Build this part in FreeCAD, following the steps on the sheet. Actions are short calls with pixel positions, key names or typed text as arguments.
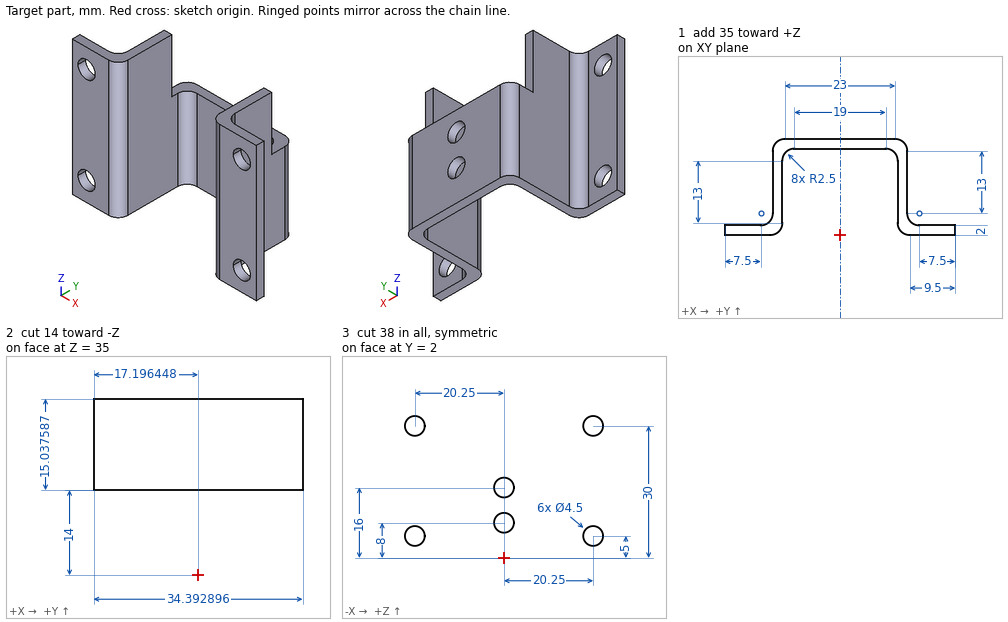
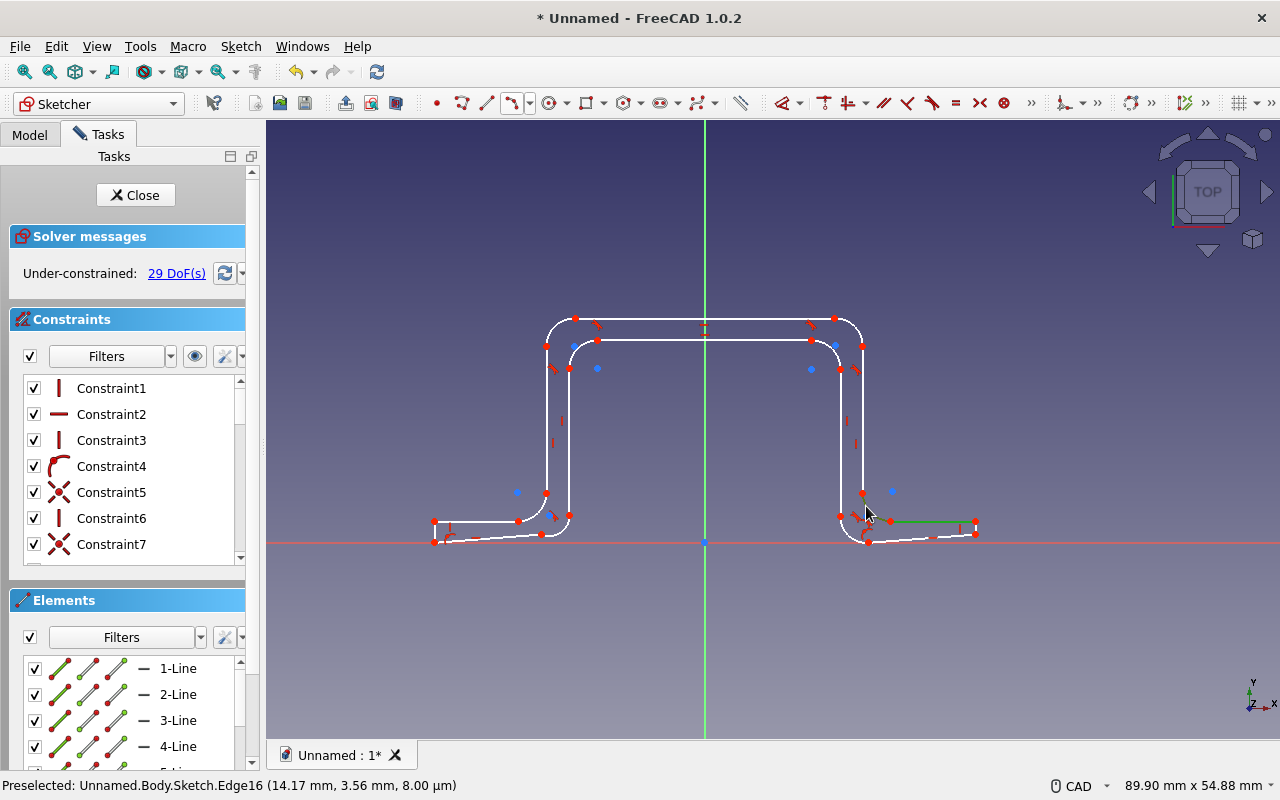
click(932, 104)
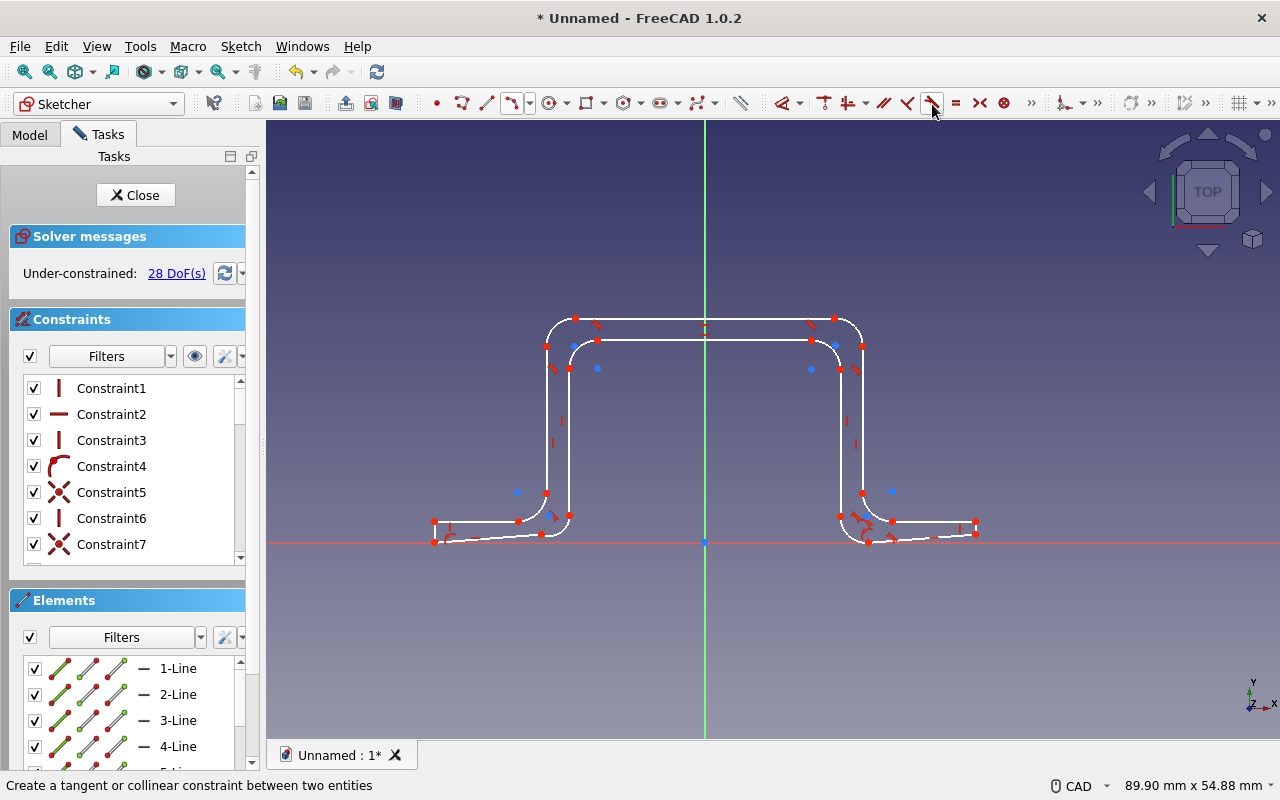
click(863, 449)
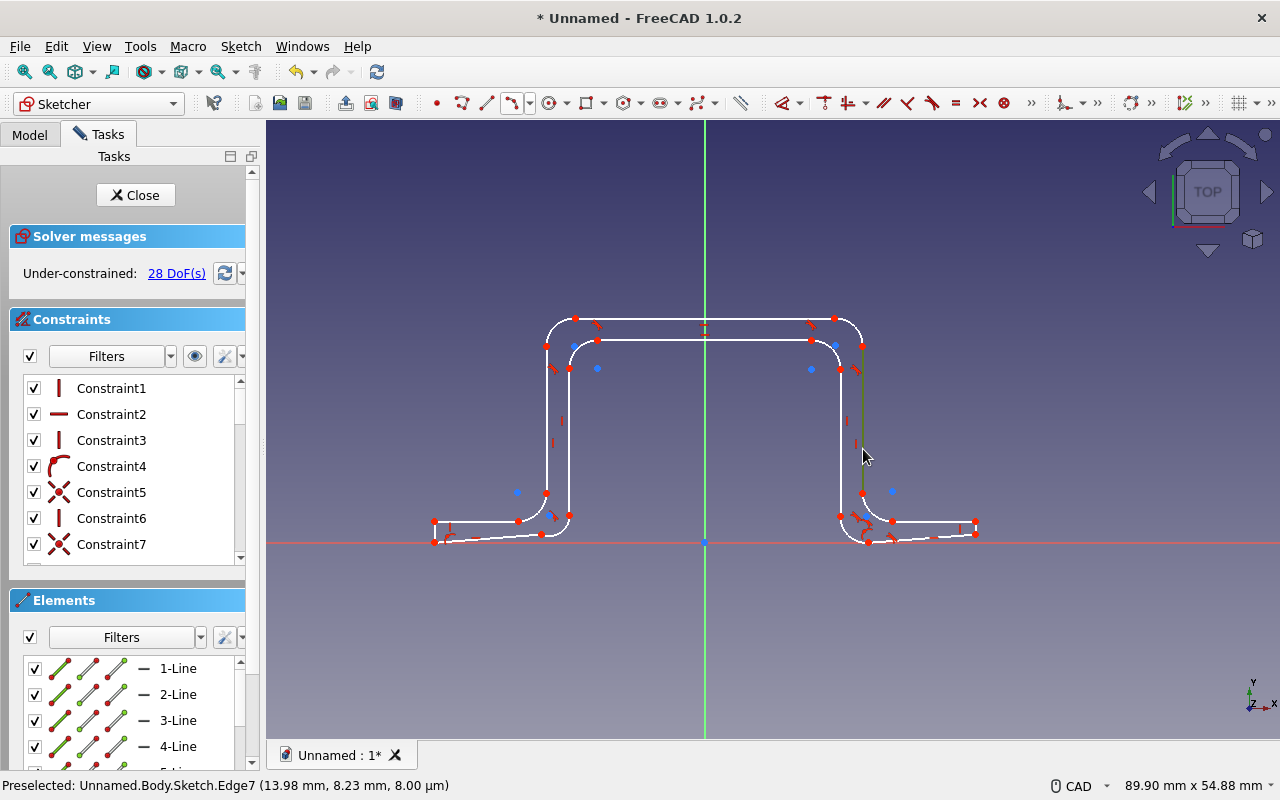
click(866, 506)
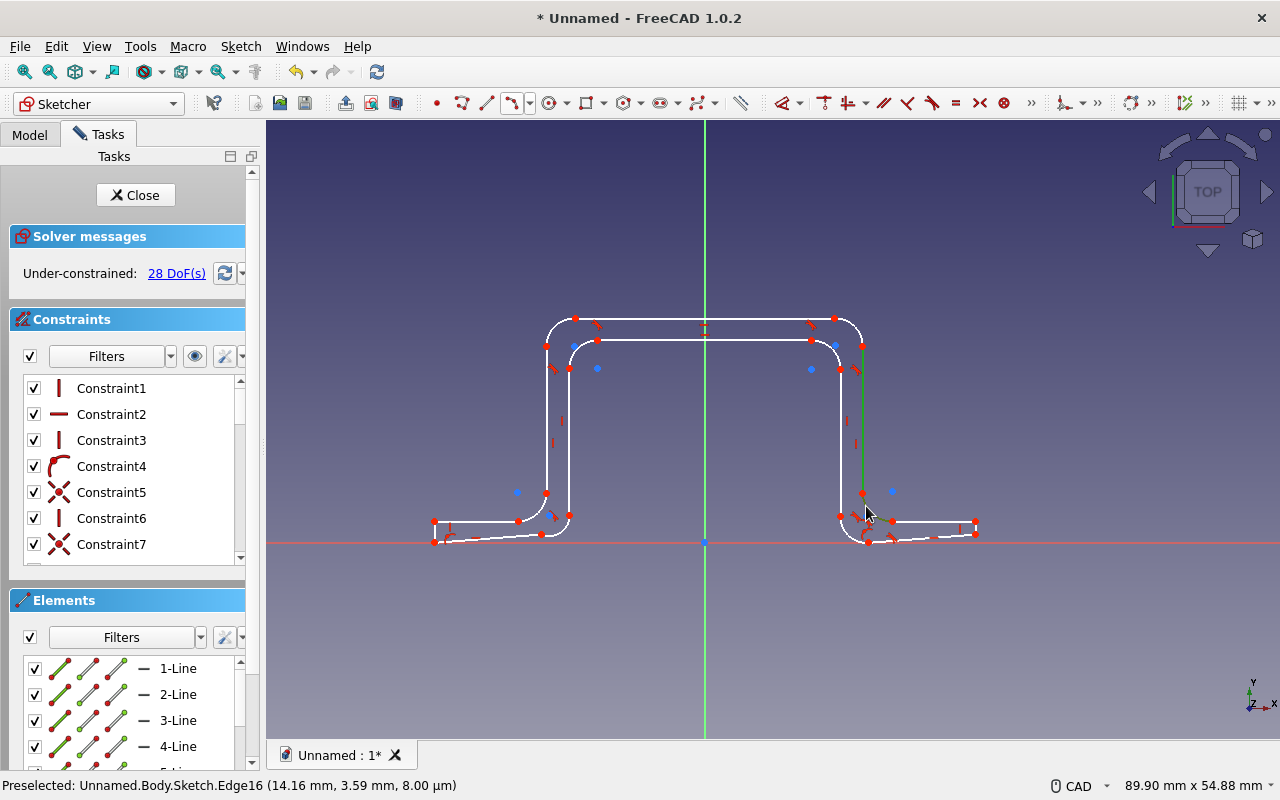
click(932, 104)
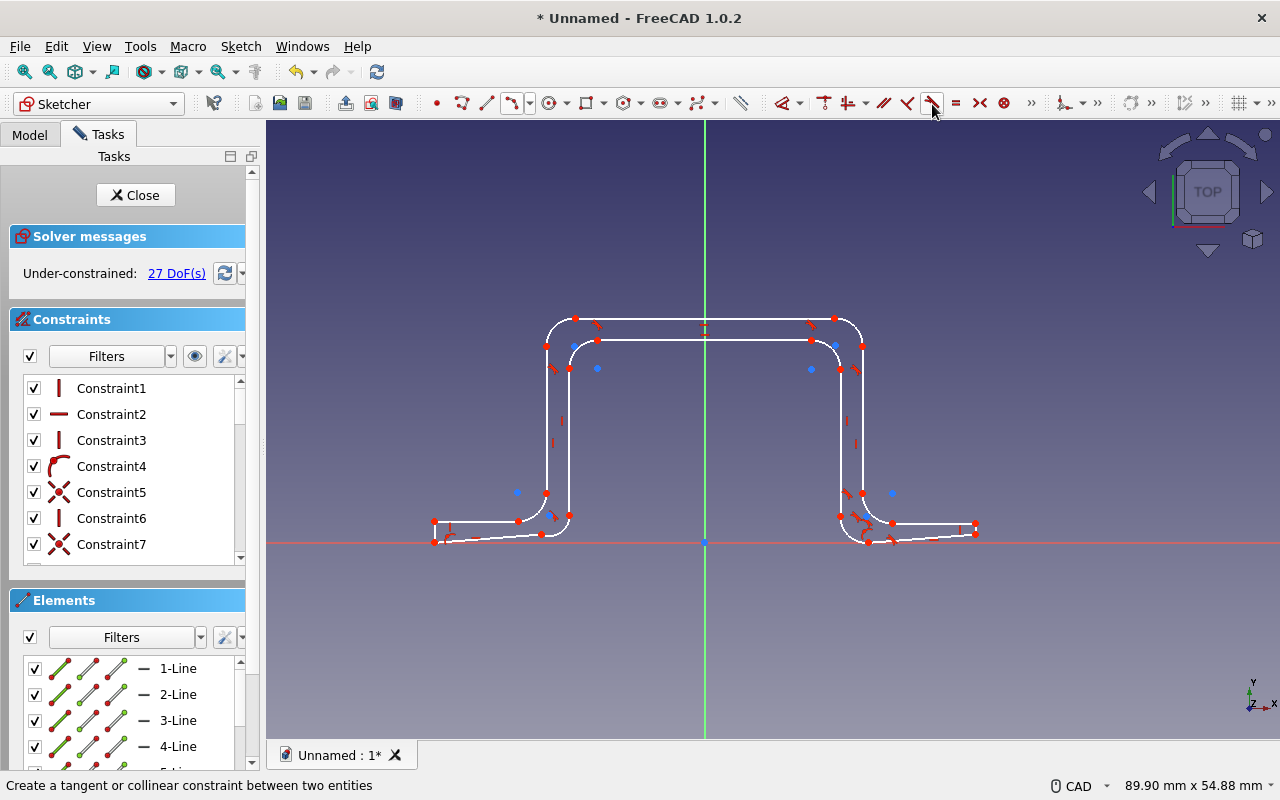
click(863, 449)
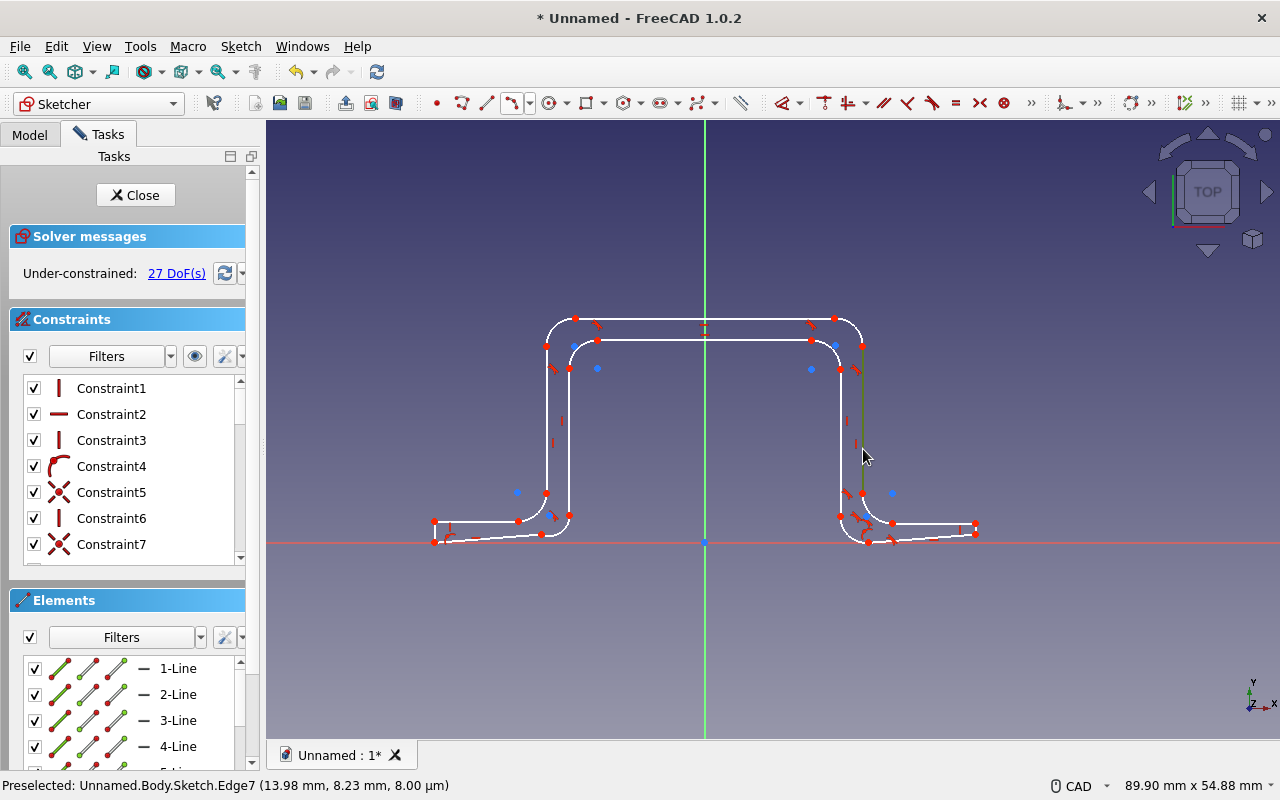
click(860, 334)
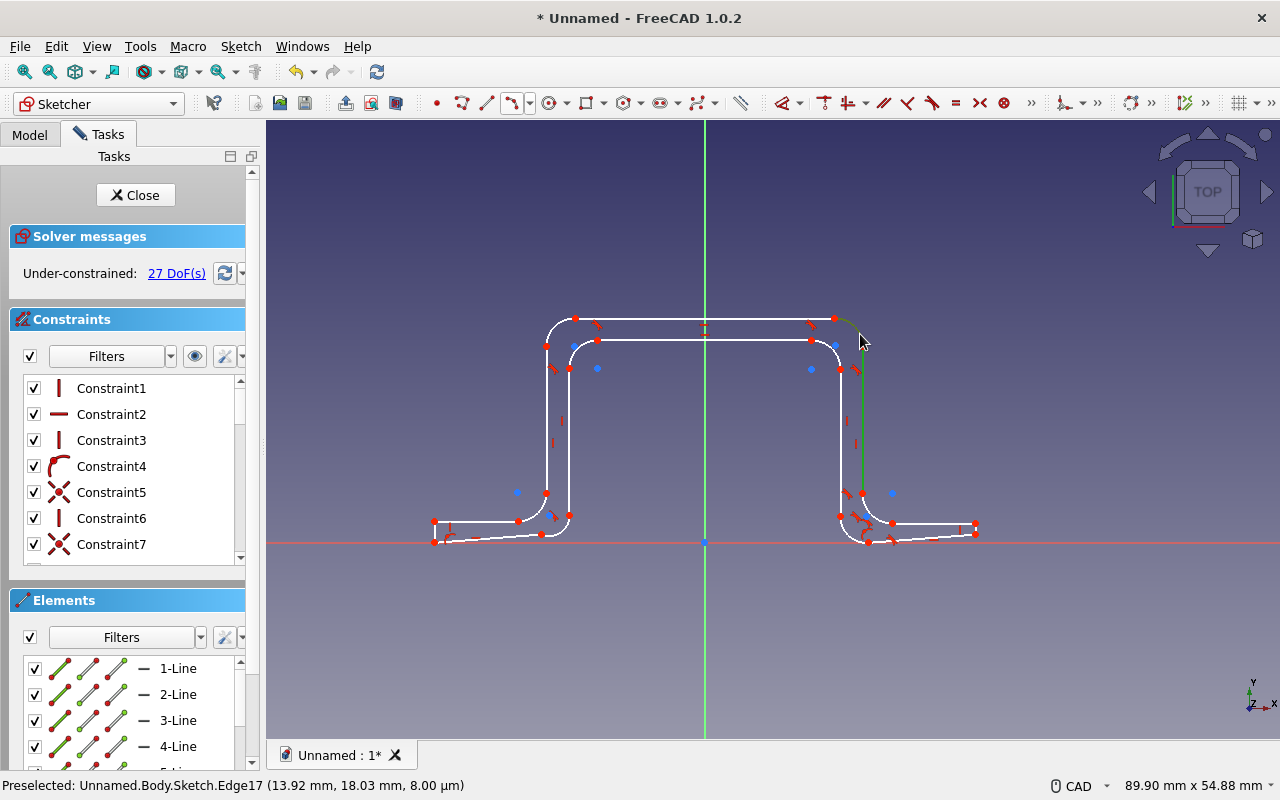
click(932, 104)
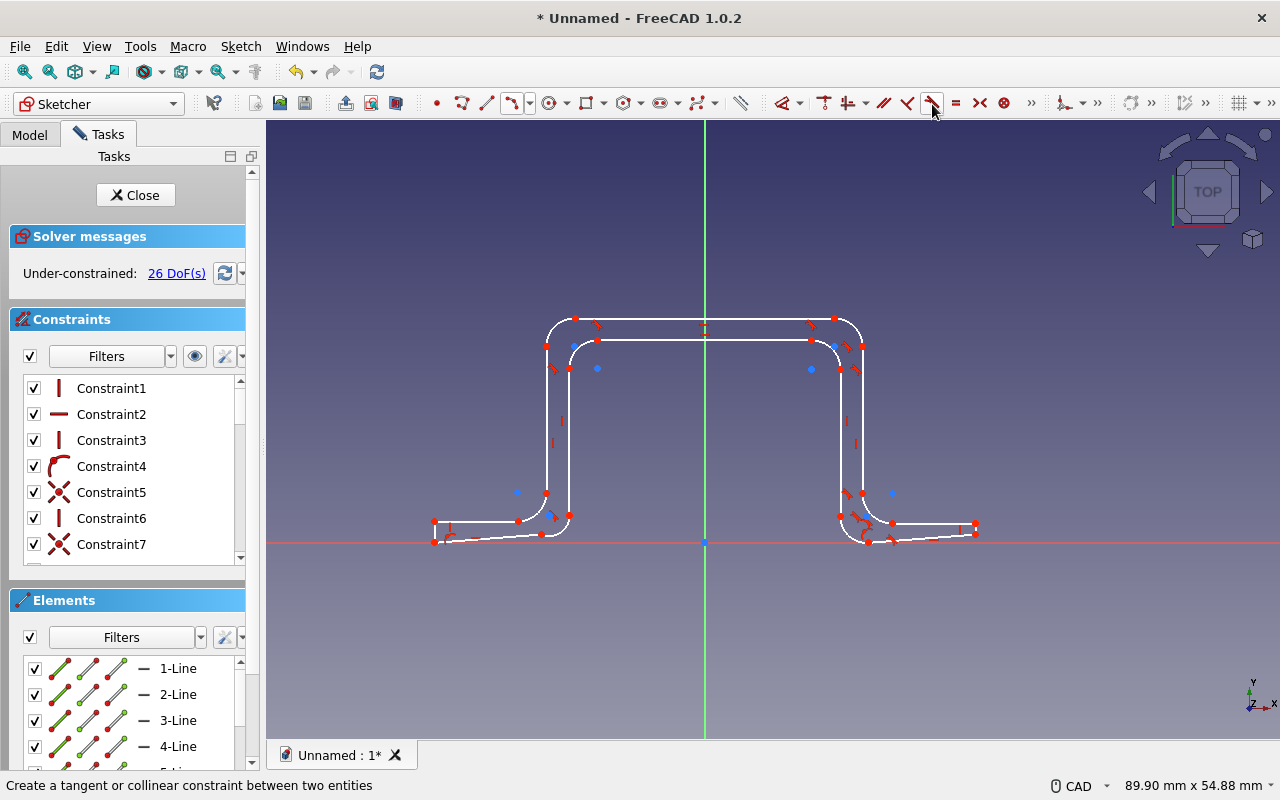
click(757, 319)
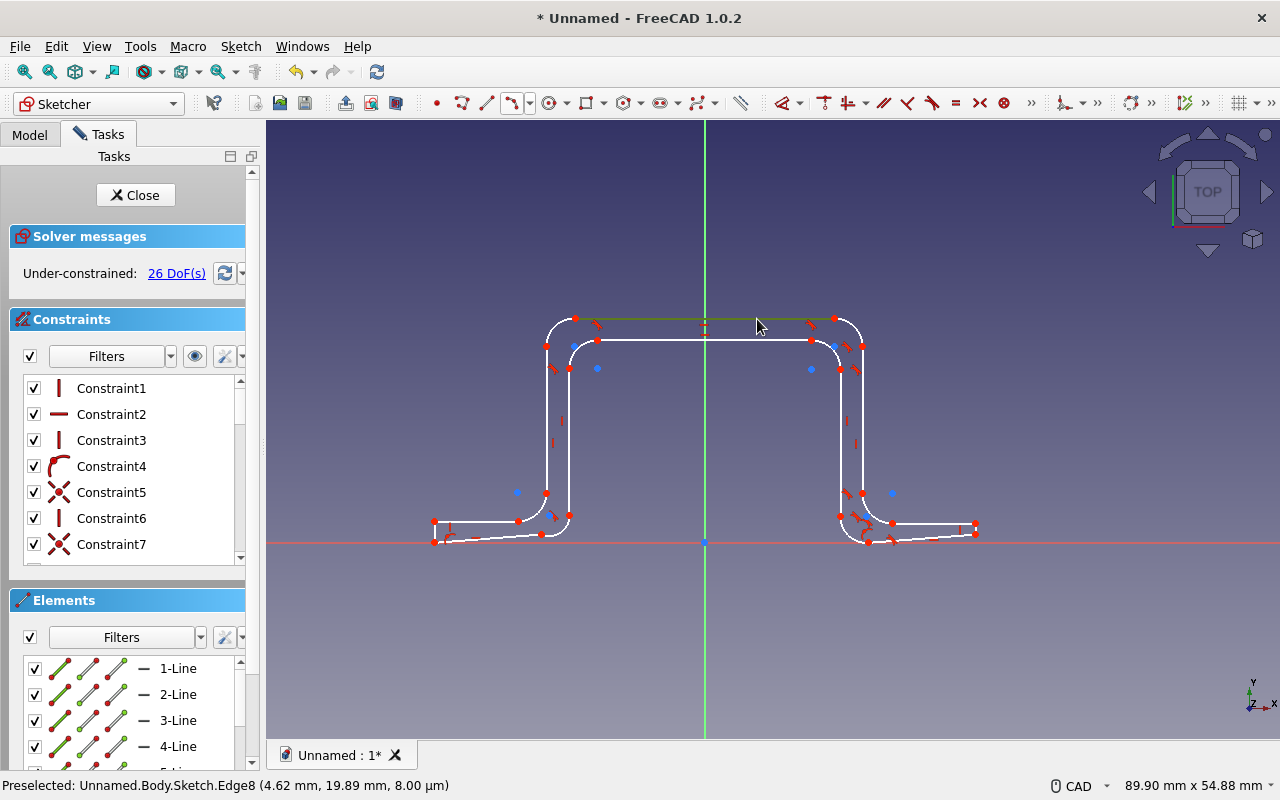
click(859, 334)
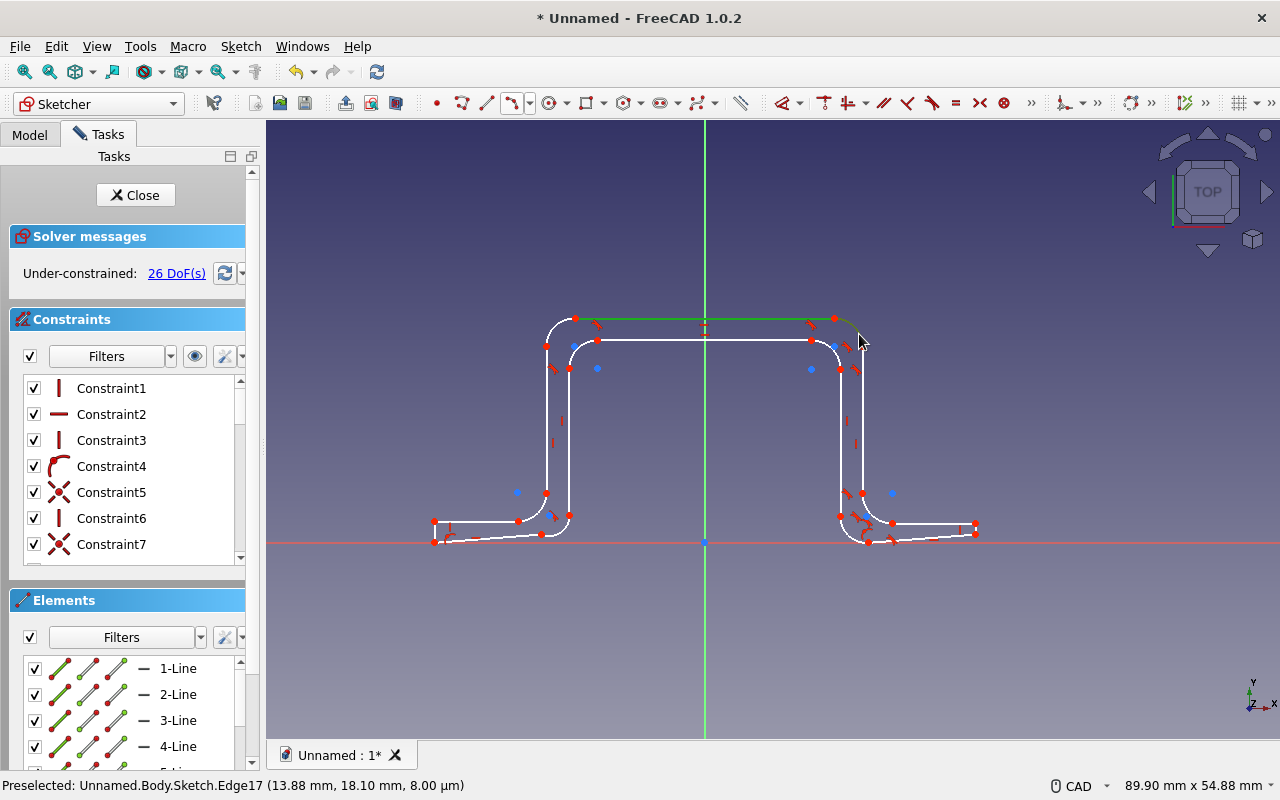
click(932, 104)